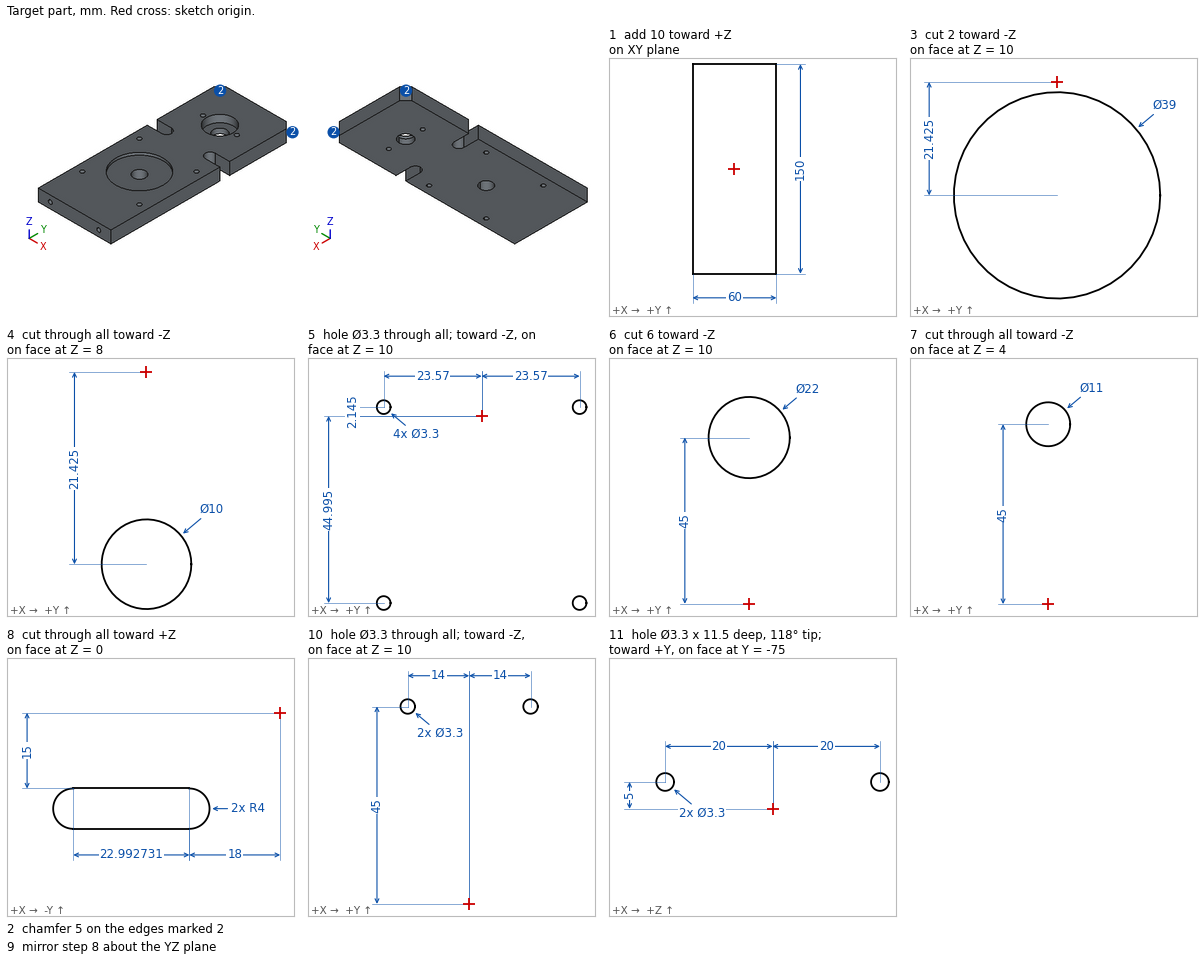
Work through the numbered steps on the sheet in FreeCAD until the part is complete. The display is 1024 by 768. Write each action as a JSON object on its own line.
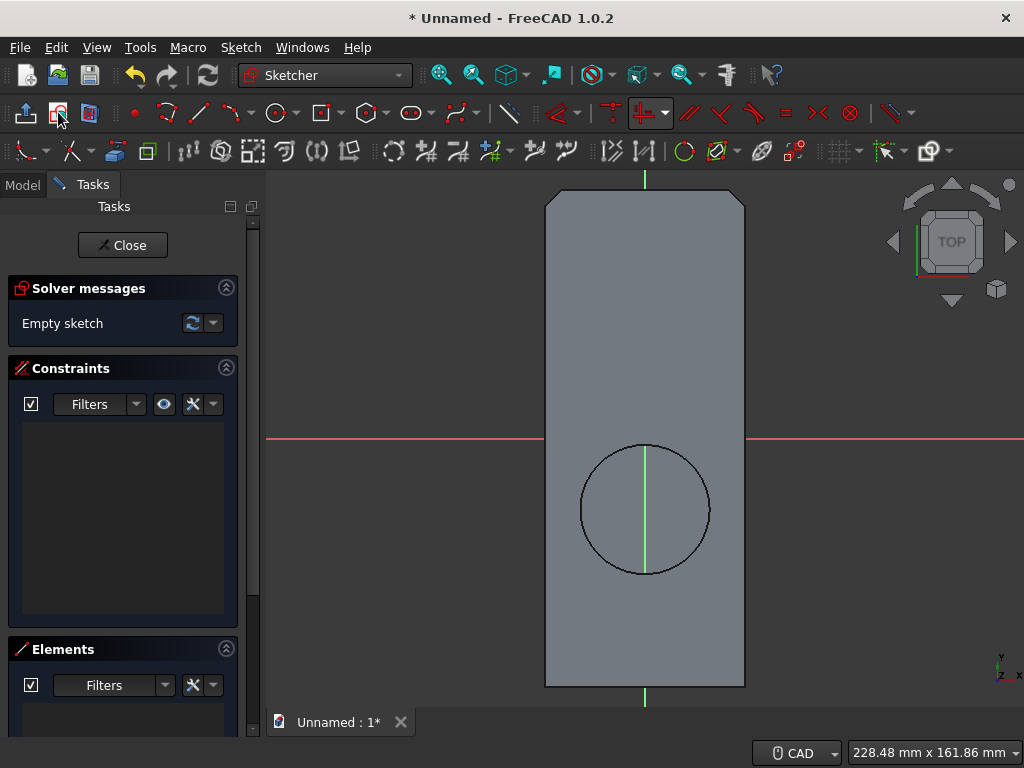
{"action": "left_click", "coordinate": [90, 114]}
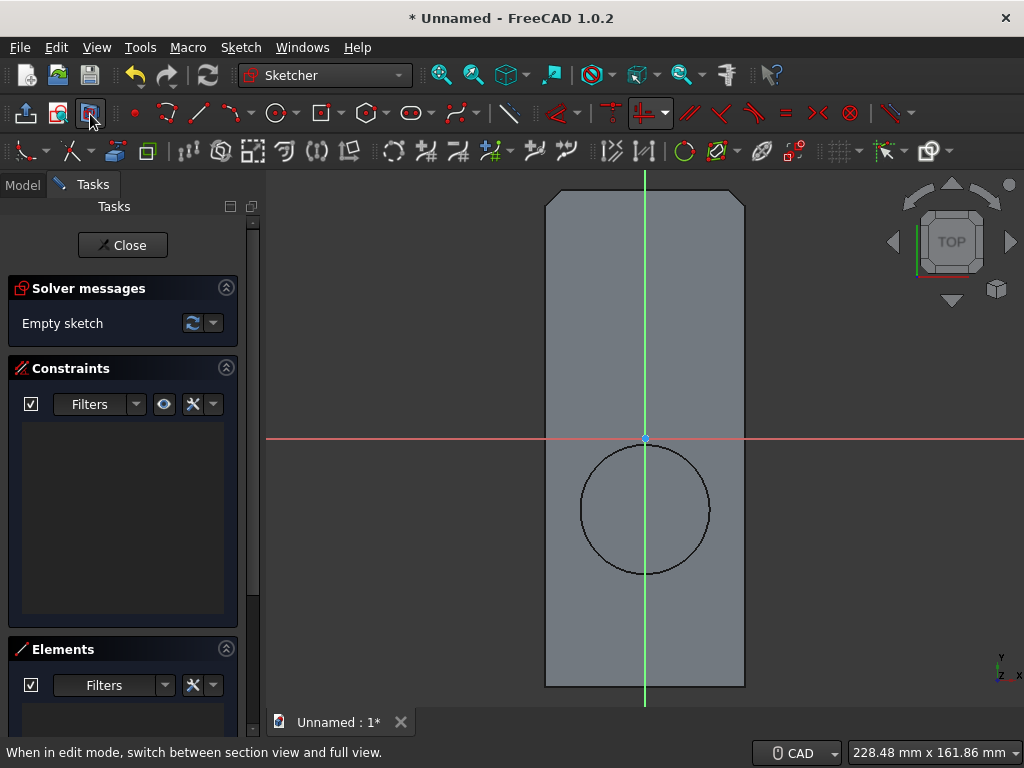
{"action": "scroll", "coordinate": [652, 517], "scroll_direction": "up", "scroll_amount": 12}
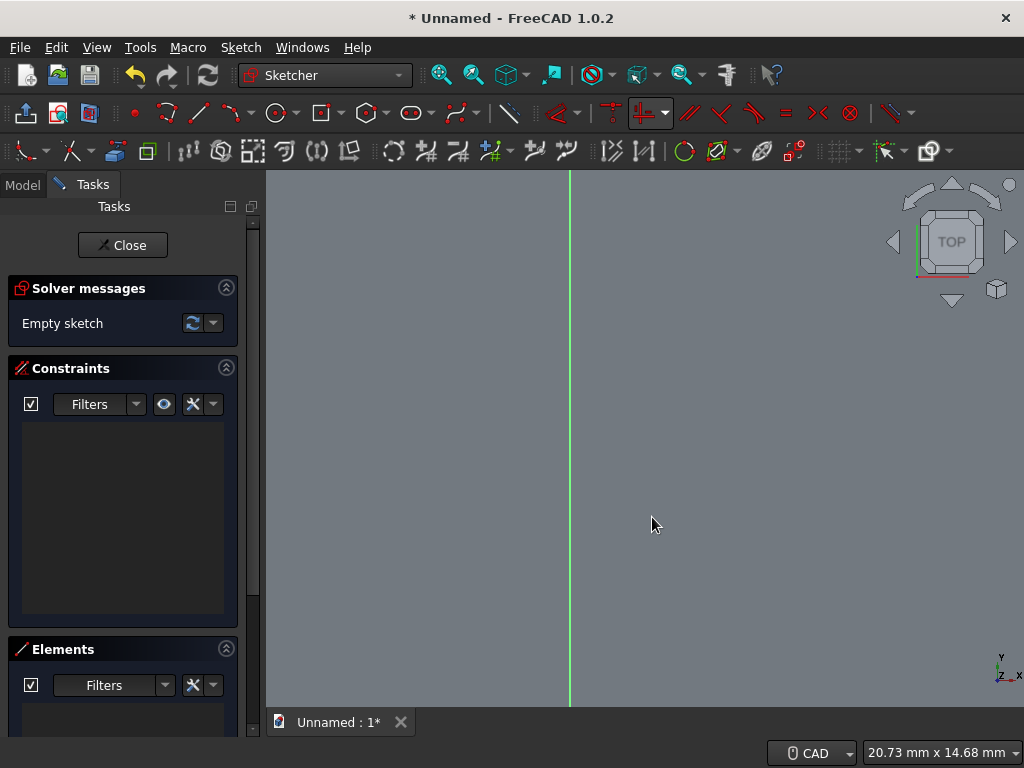
{"action": "left_click", "coordinate": [276, 114]}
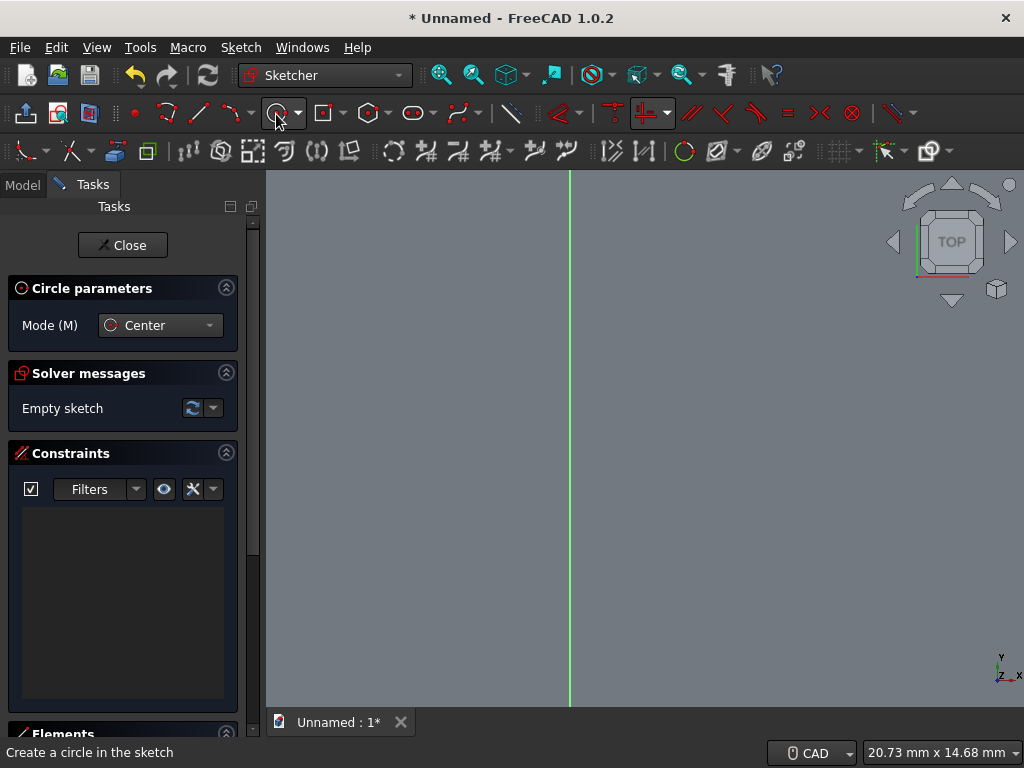
{"action": "left_click", "coordinate": [570, 429]}
{"action": "left_click", "coordinate": [699, 299]}
{"action": "key", "text": "Escape"}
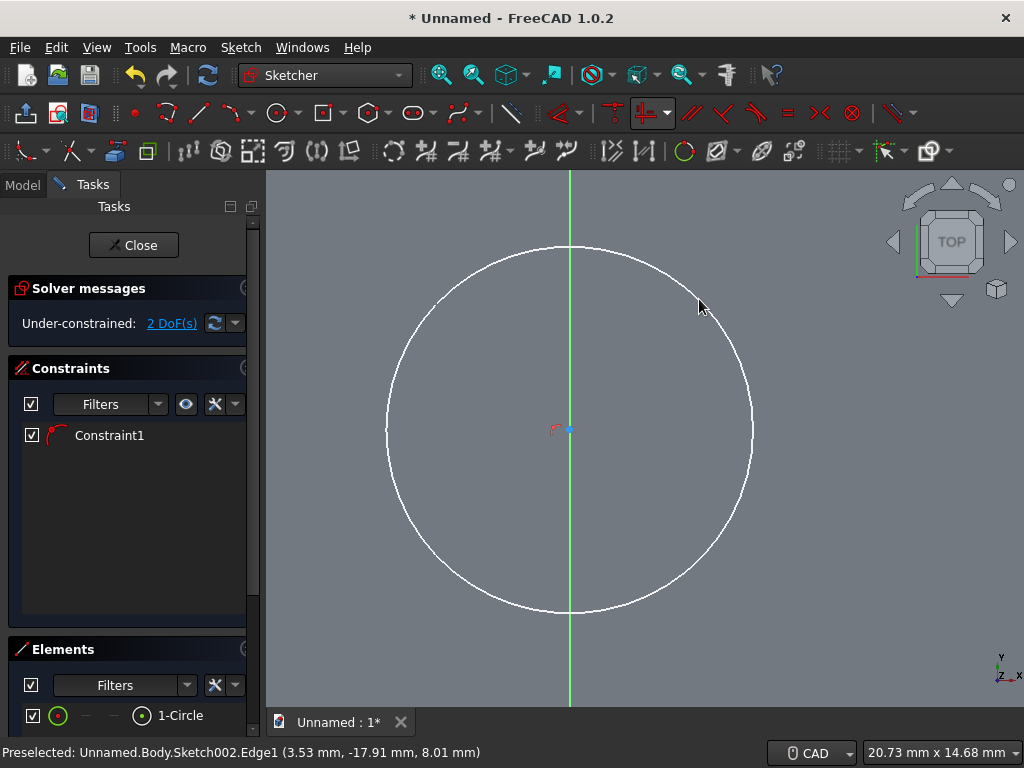
{"action": "left_click", "coordinate": [558, 114]}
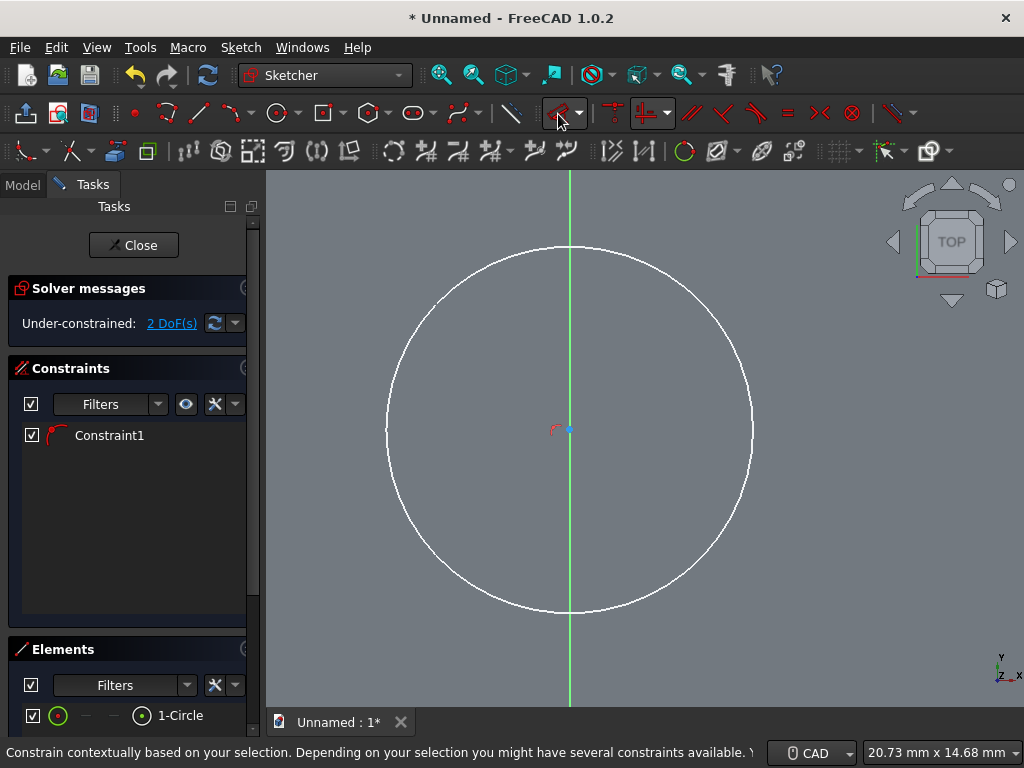
{"action": "left_click", "coordinate": [699, 300]}
{"action": "left_click", "coordinate": [722, 277]}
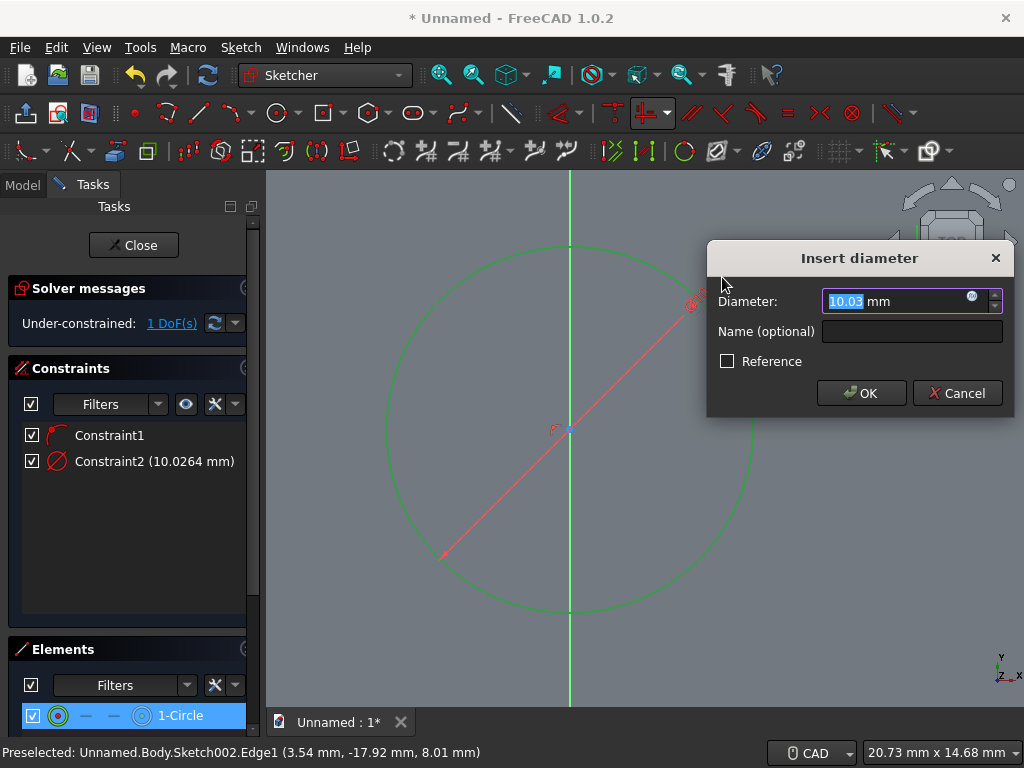
{"action": "type", "text": "10"}
{"action": "key", "text": "Return"}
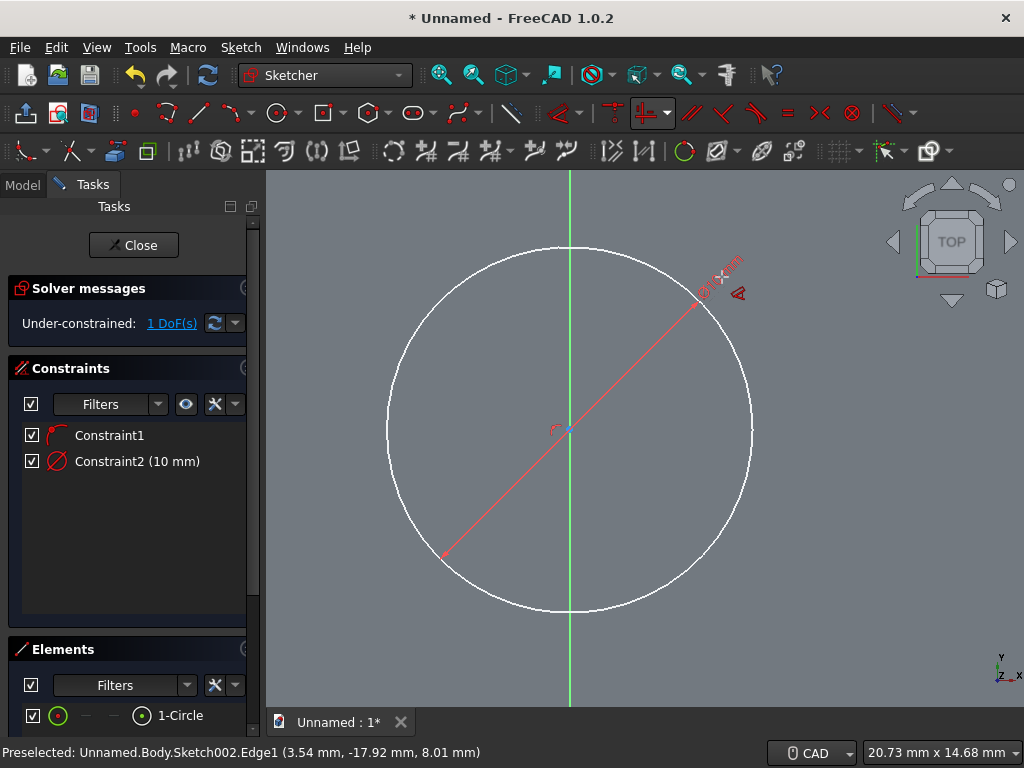
{"action": "left_click", "coordinate": [570, 430]}
{"action": "left_click", "coordinate": [604, 314]}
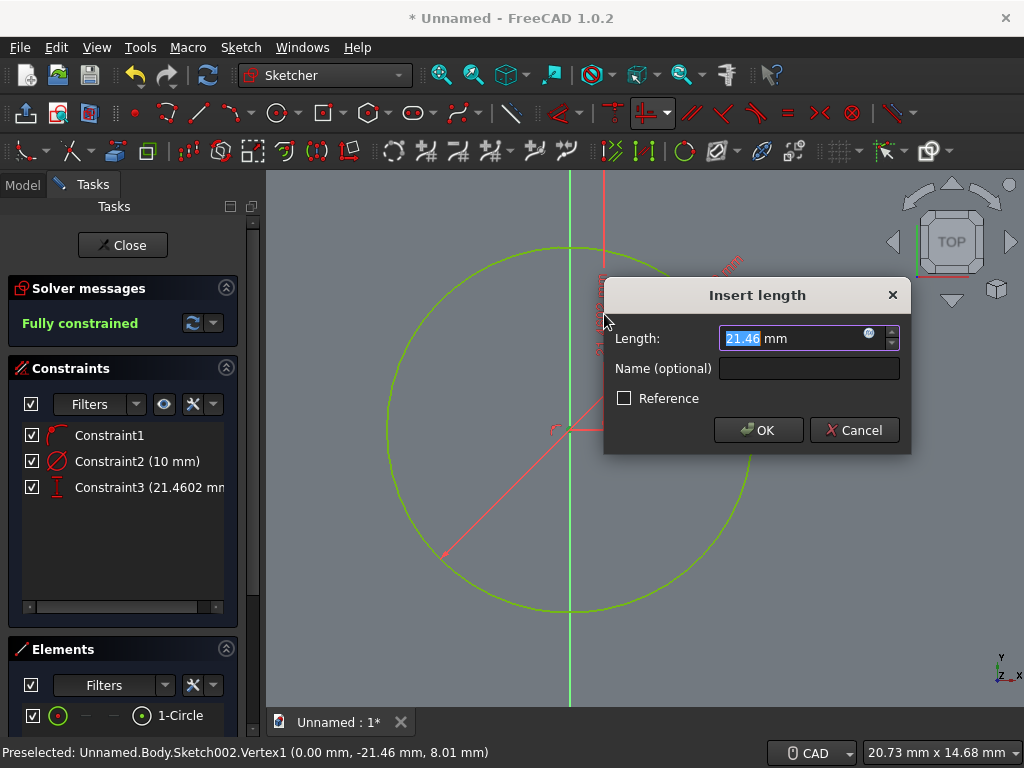
{"action": "type", "text": "21.425"}
{"action": "key", "text": "Return"}
{"action": "key", "text": "Escape"}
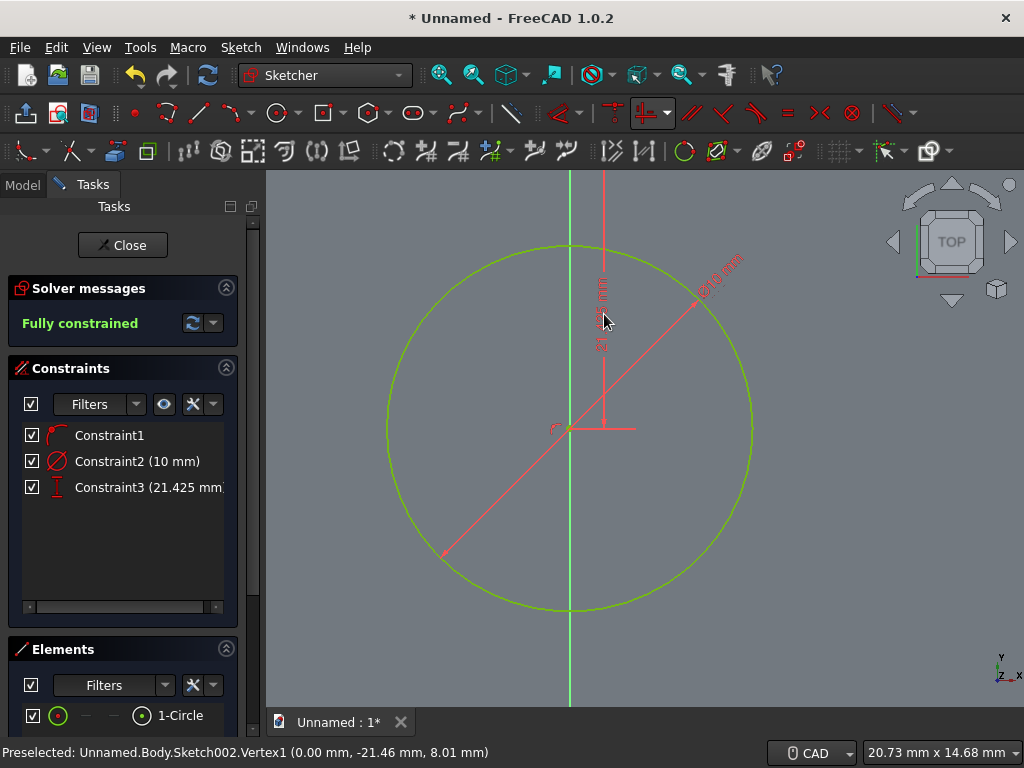
{"action": "left_click", "coordinate": [123, 245]}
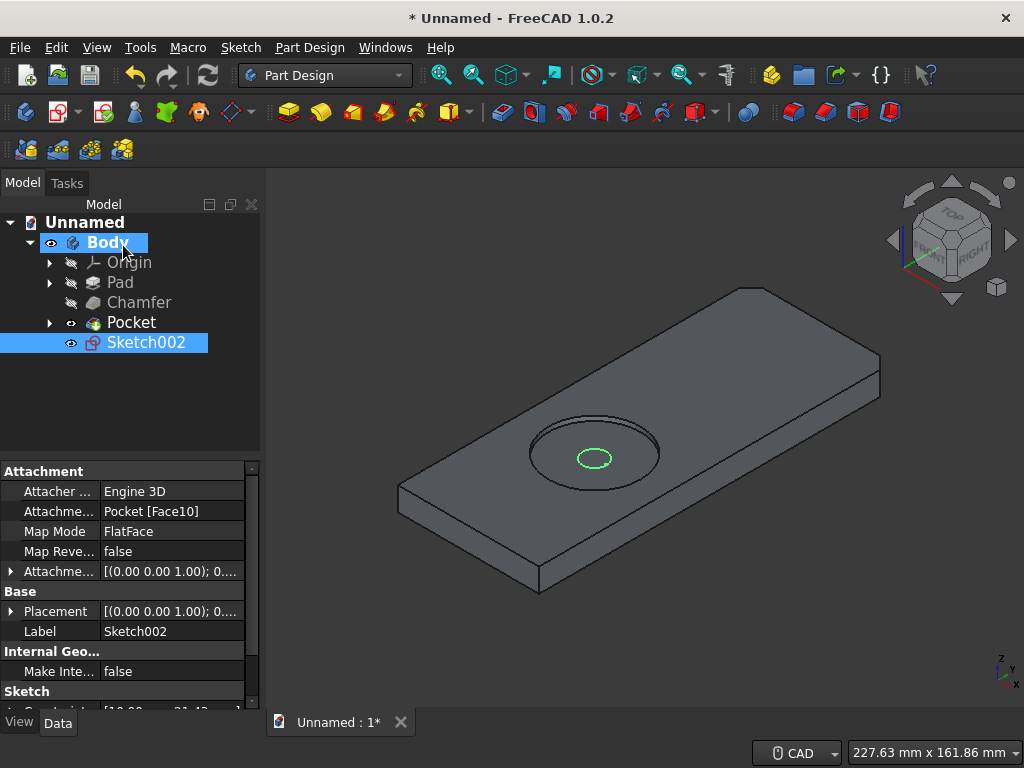
{"action": "left_click", "coordinate": [504, 112]}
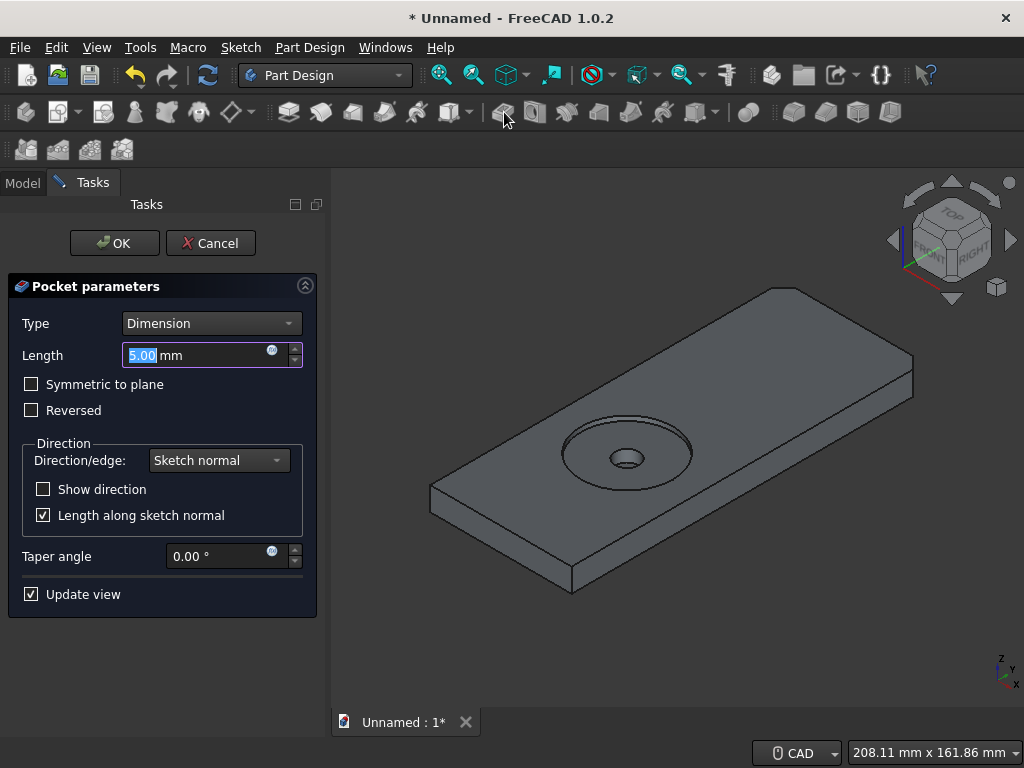
{"action": "left_click", "coordinate": [212, 324]}